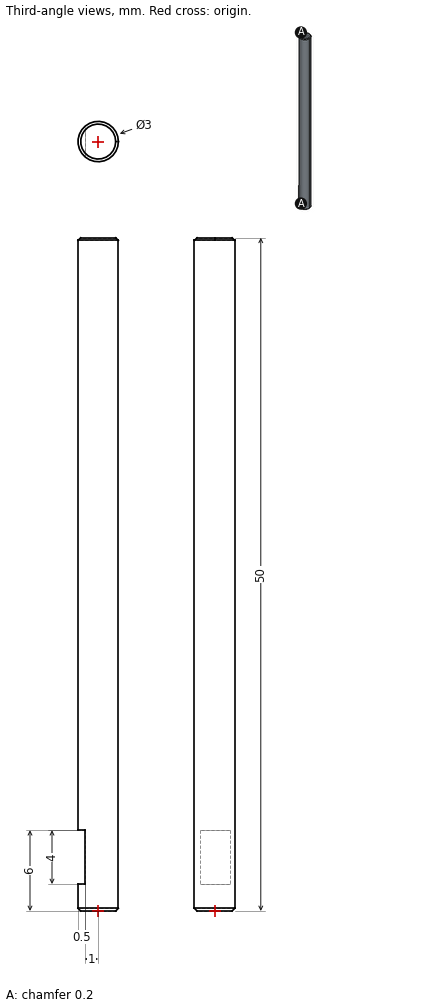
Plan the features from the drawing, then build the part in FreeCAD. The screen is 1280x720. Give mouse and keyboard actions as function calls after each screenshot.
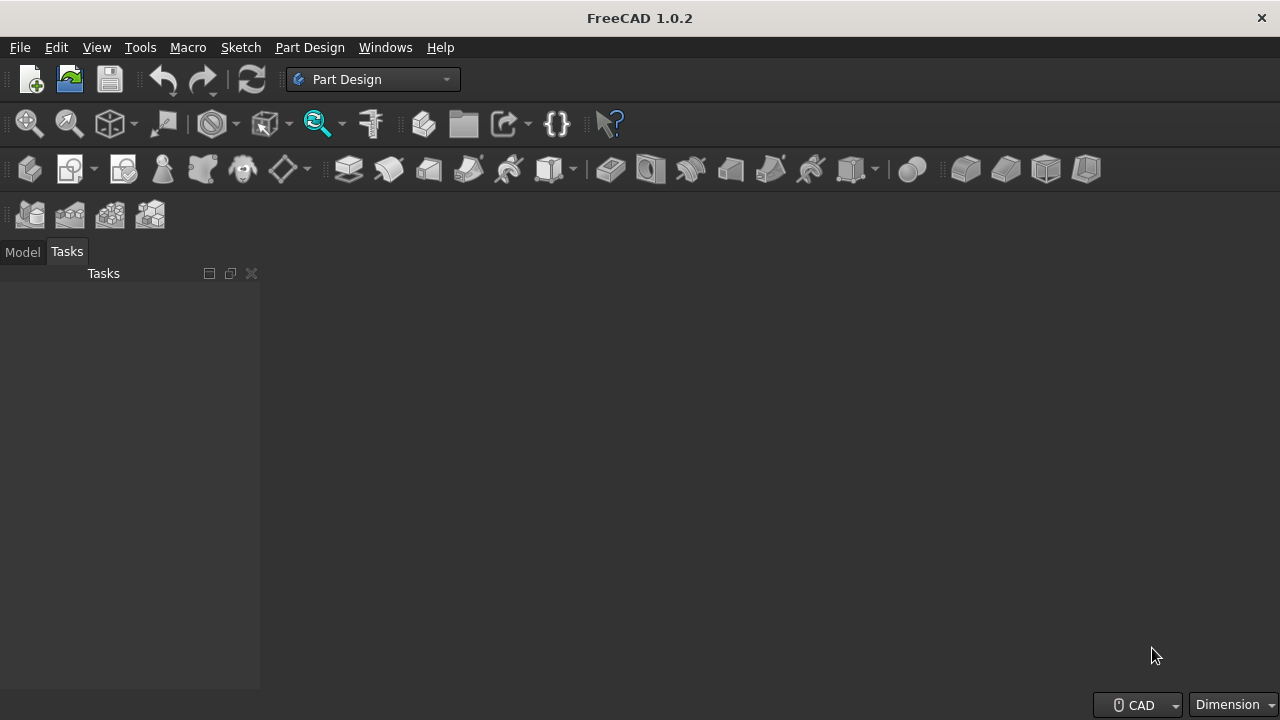
click(30, 80)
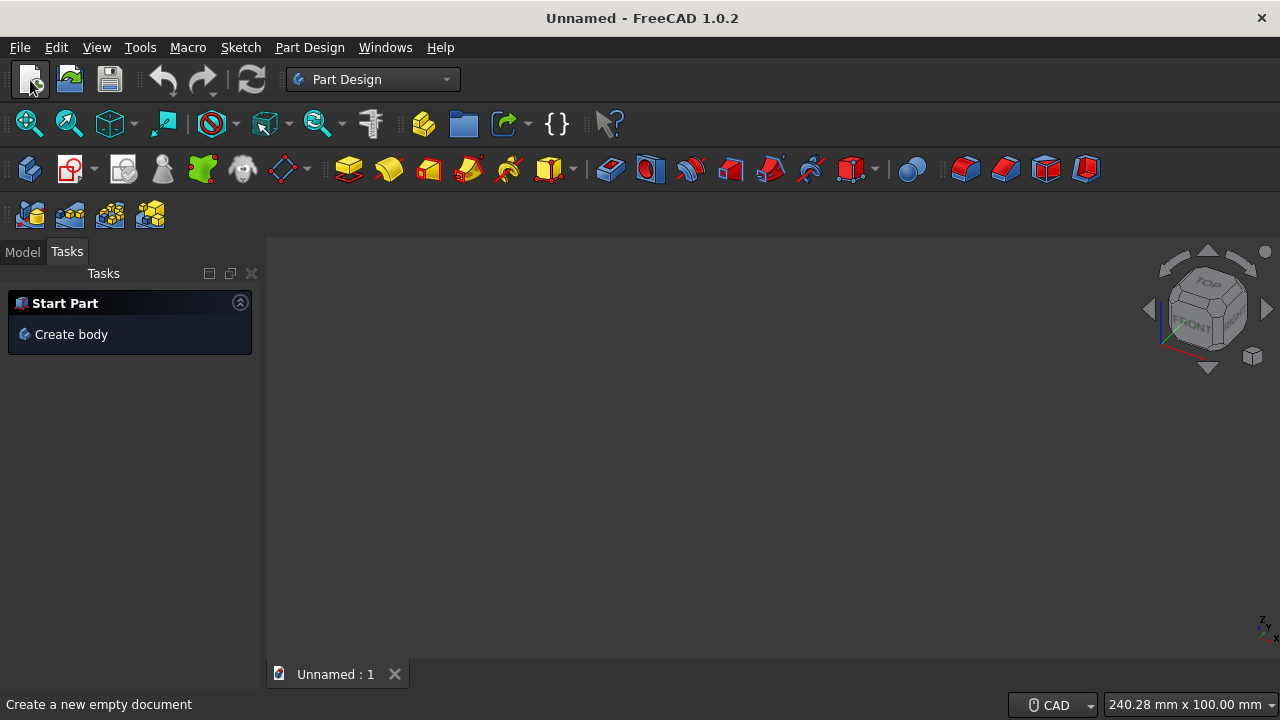
click(70, 170)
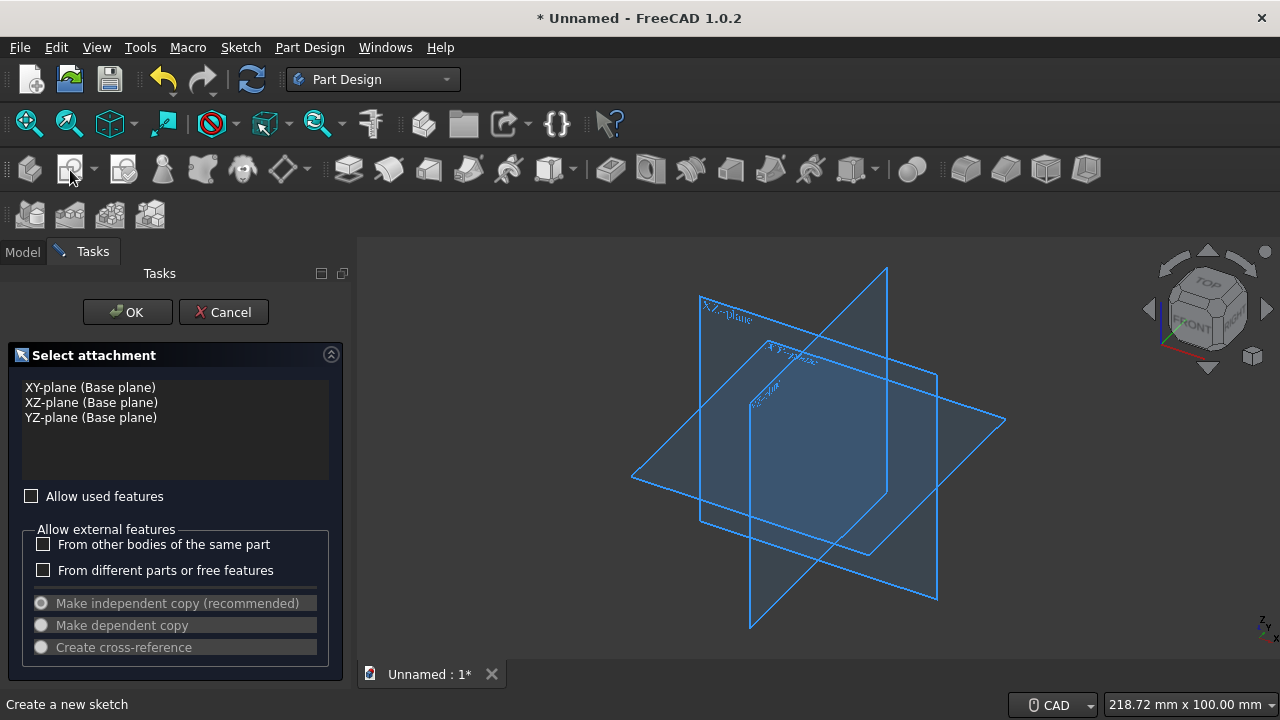
click(82, 388)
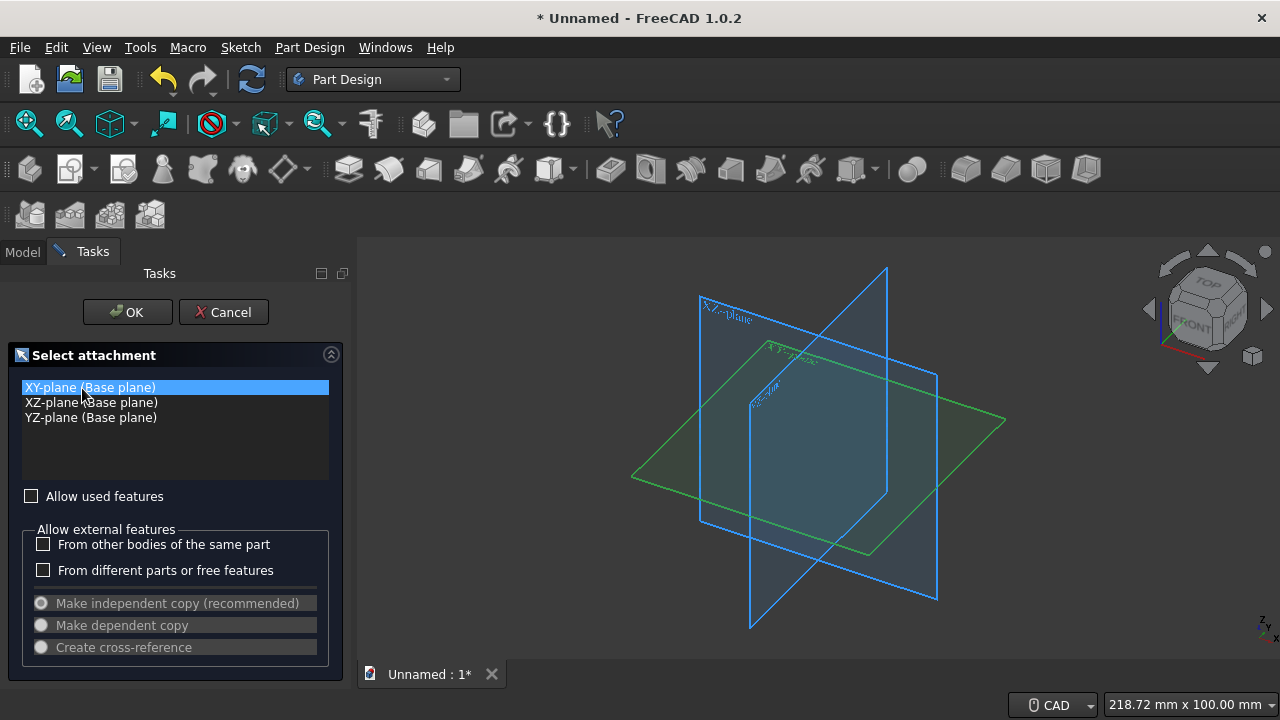
click(128, 312)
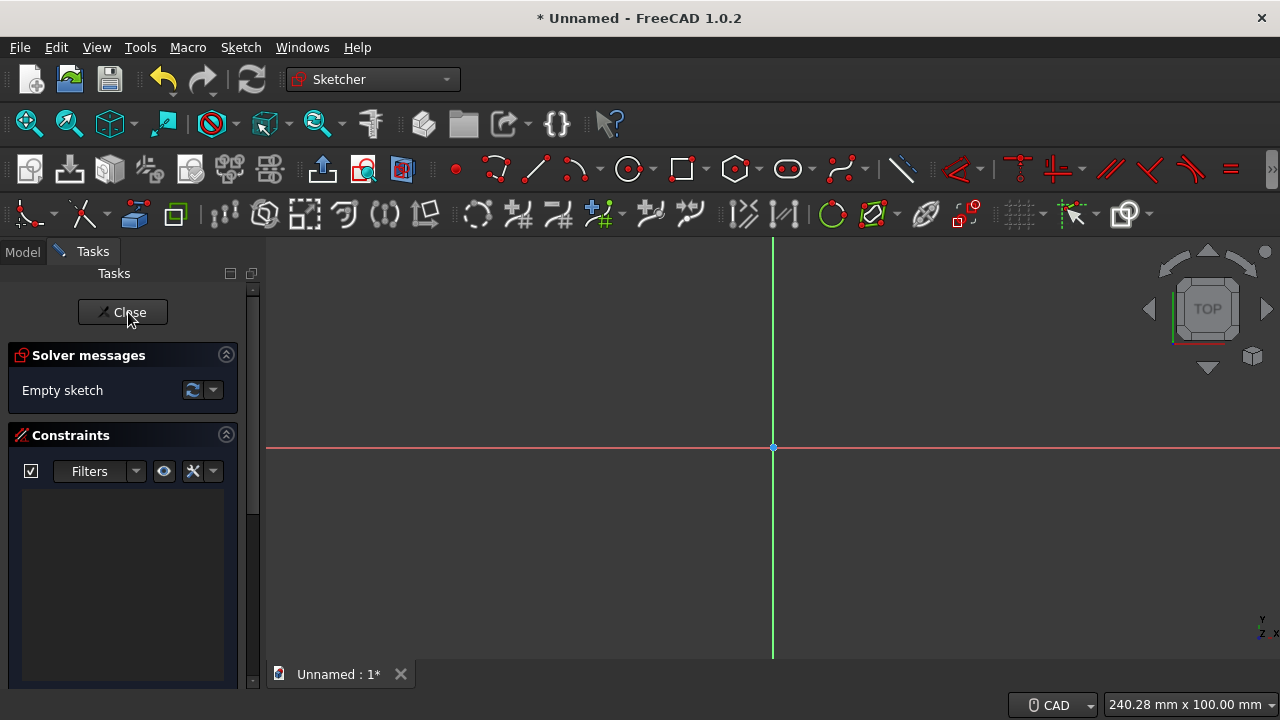
scroll(777, 448, up, 15)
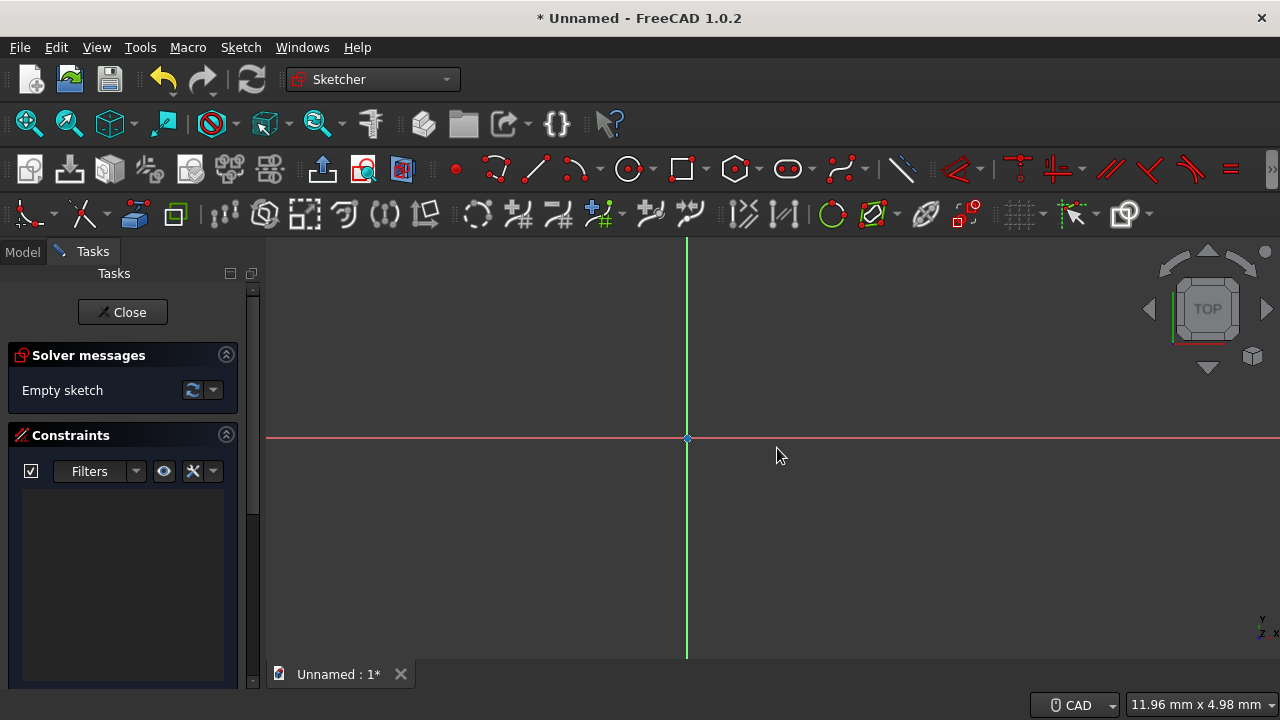
click(630, 170)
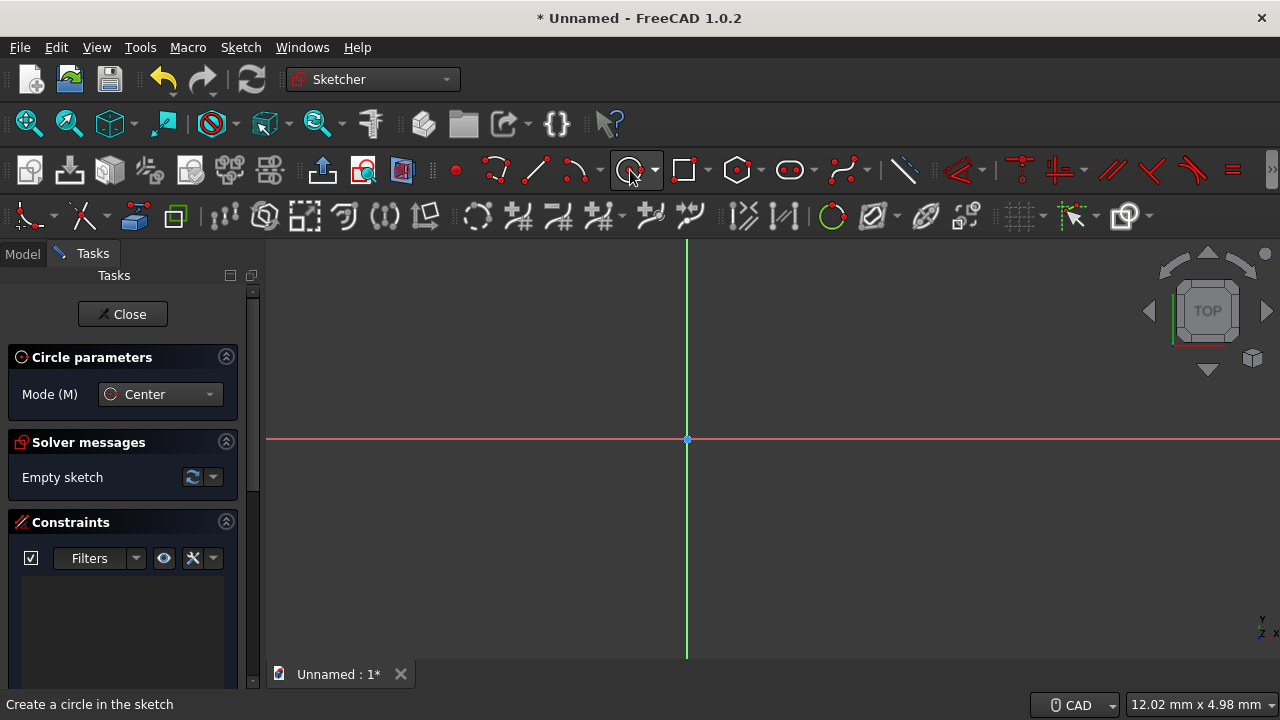
click(687, 439)
click(777, 350)
key(Escape)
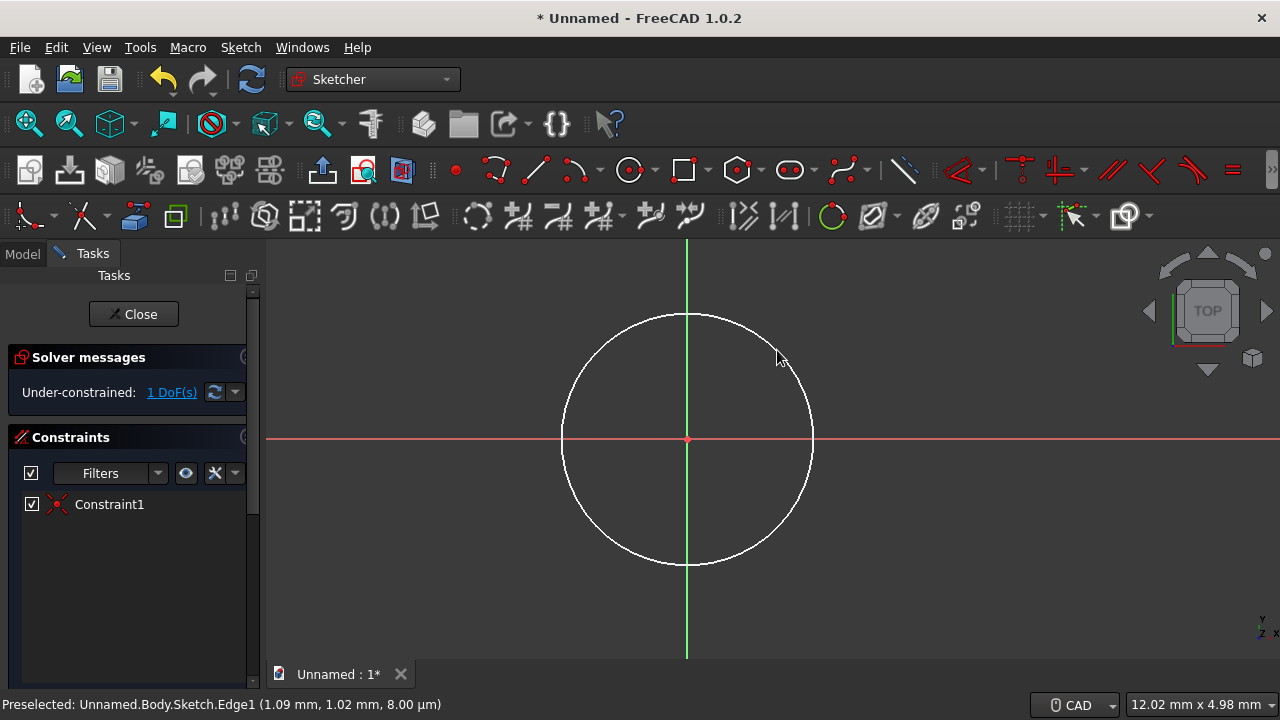
click(958, 170)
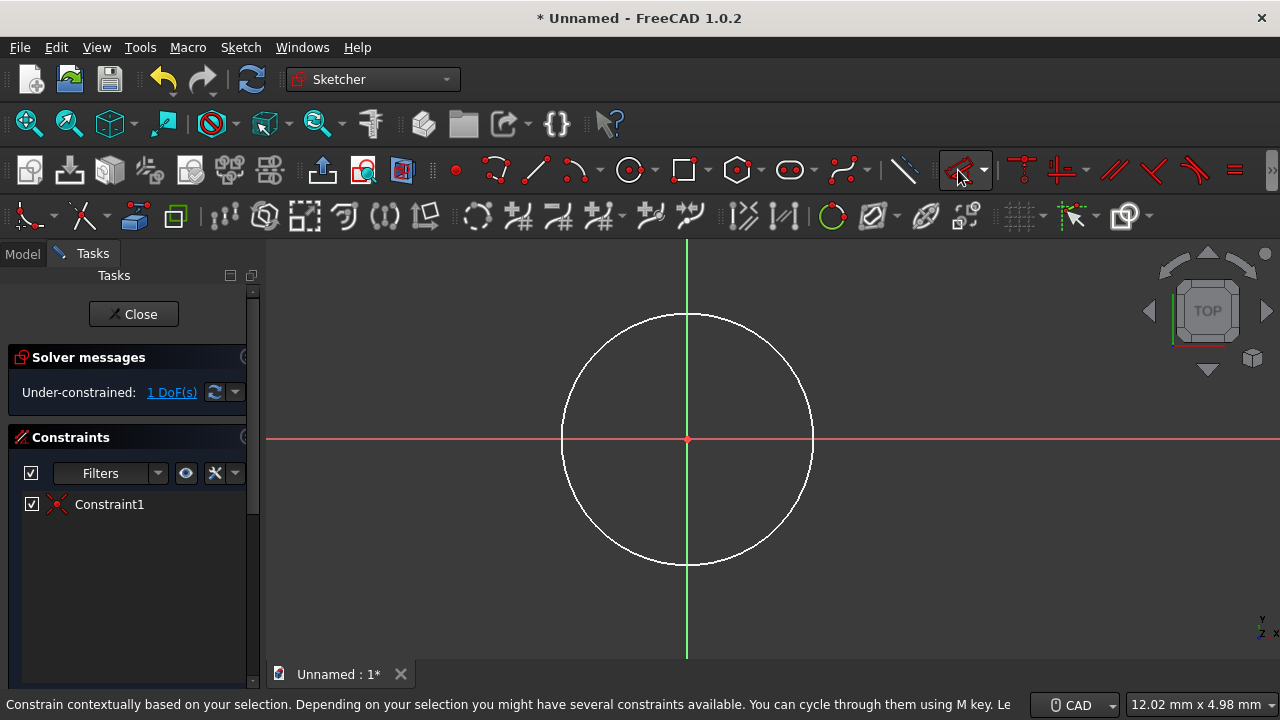
click(776, 350)
click(799, 327)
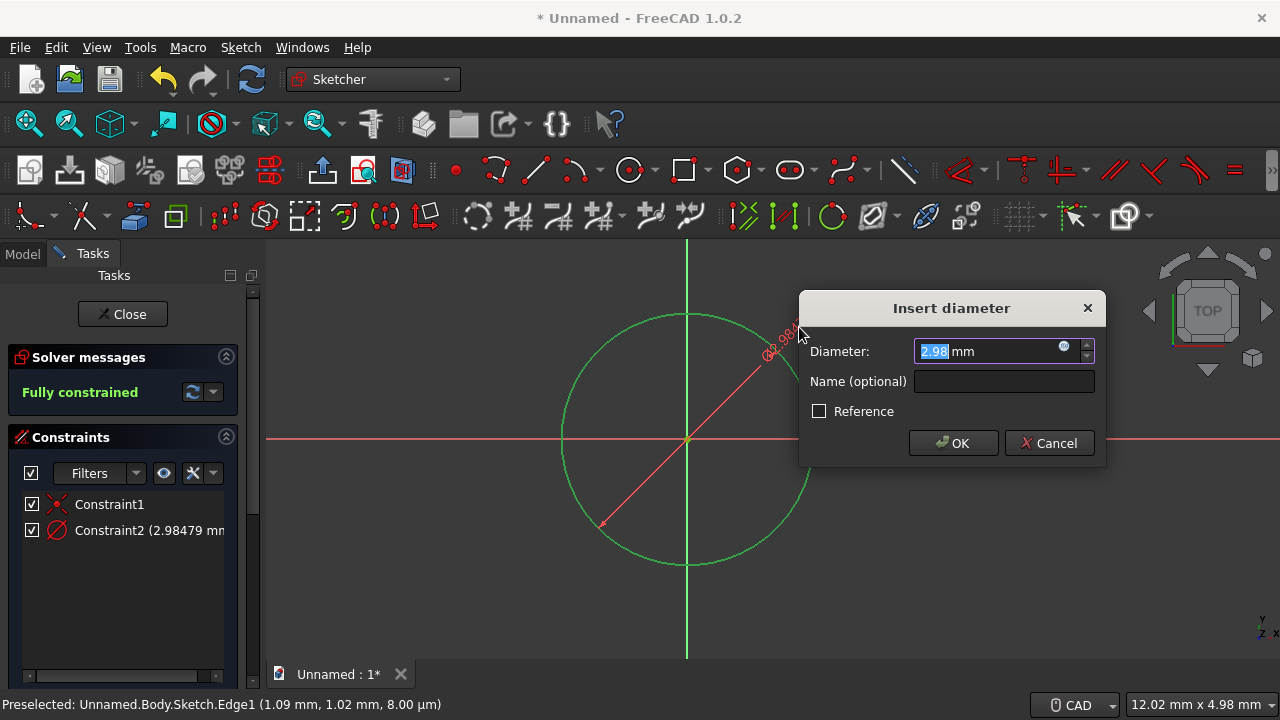
text(3)
key(Return)
key(Escape)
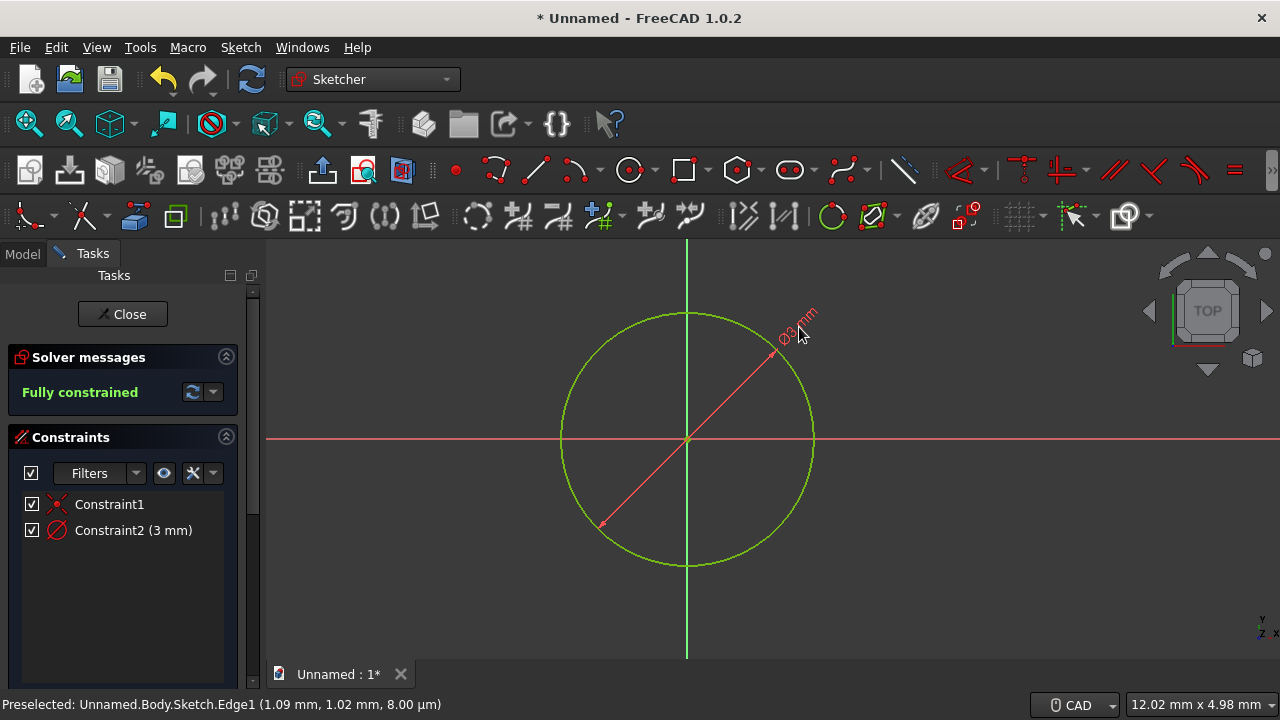
click(123, 314)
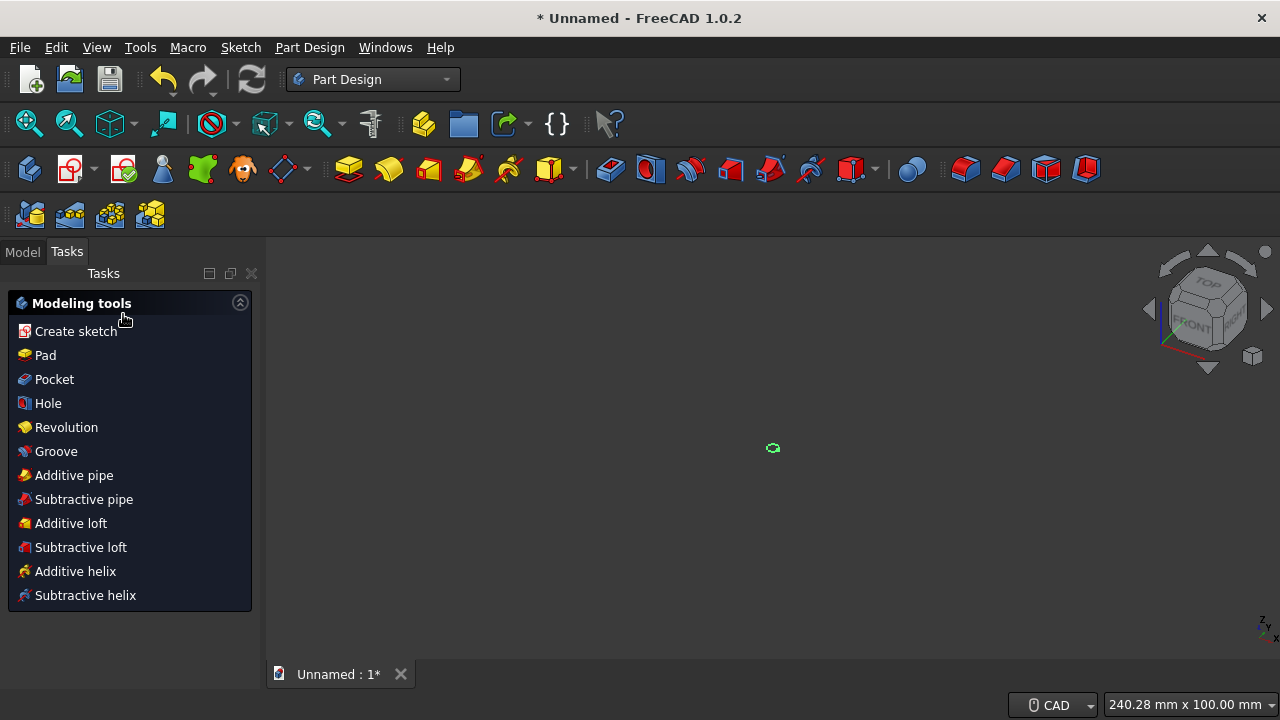
click(350, 170)